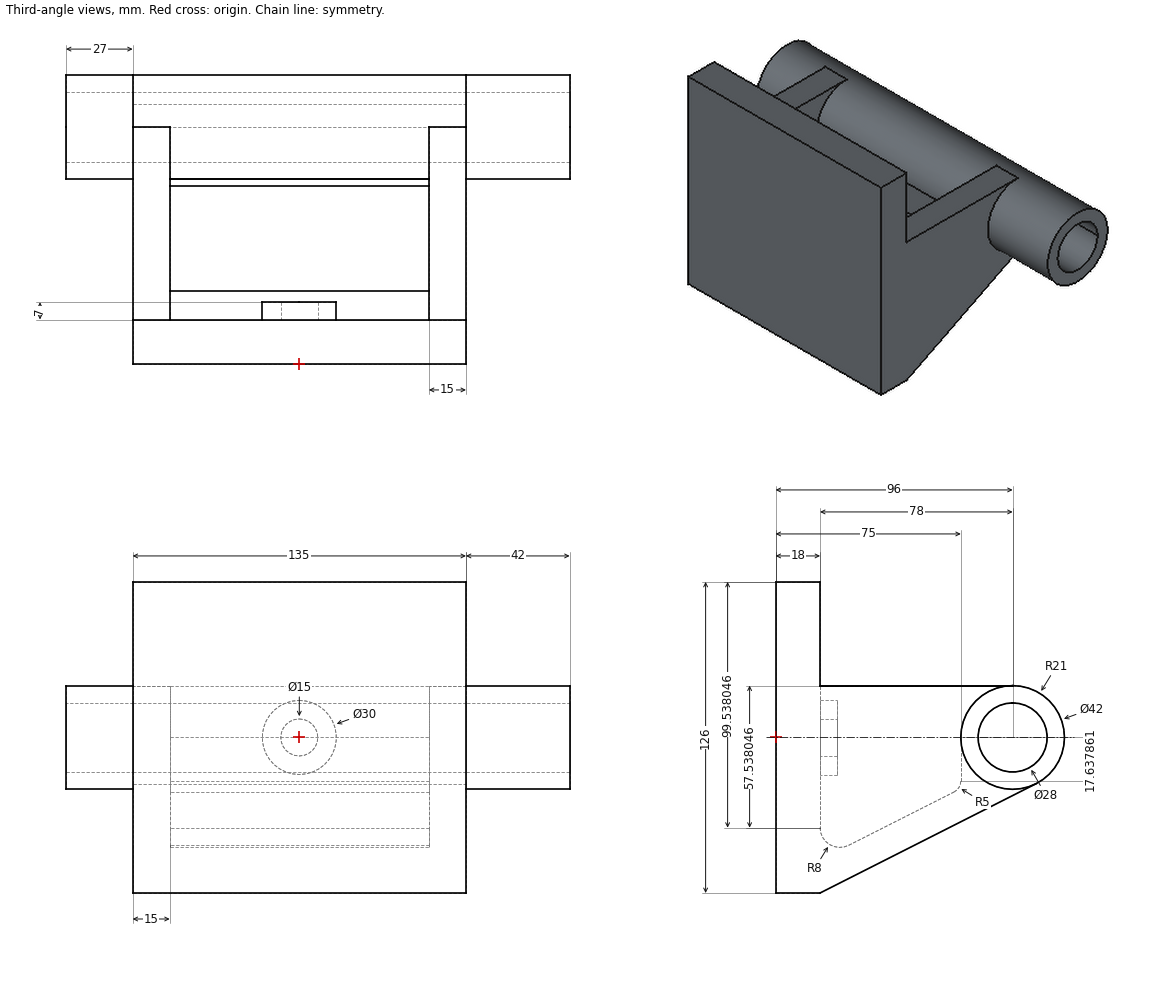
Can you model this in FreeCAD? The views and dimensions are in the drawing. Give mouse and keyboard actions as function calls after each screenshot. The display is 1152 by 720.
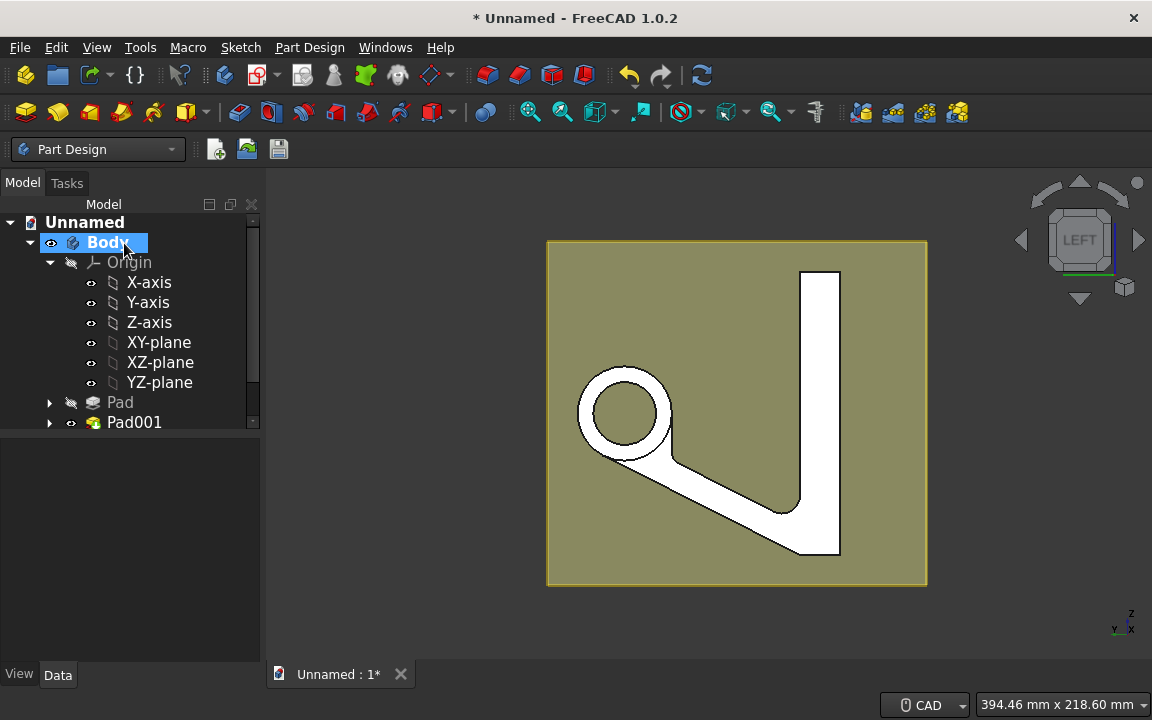
scroll(100, 318, down, 3)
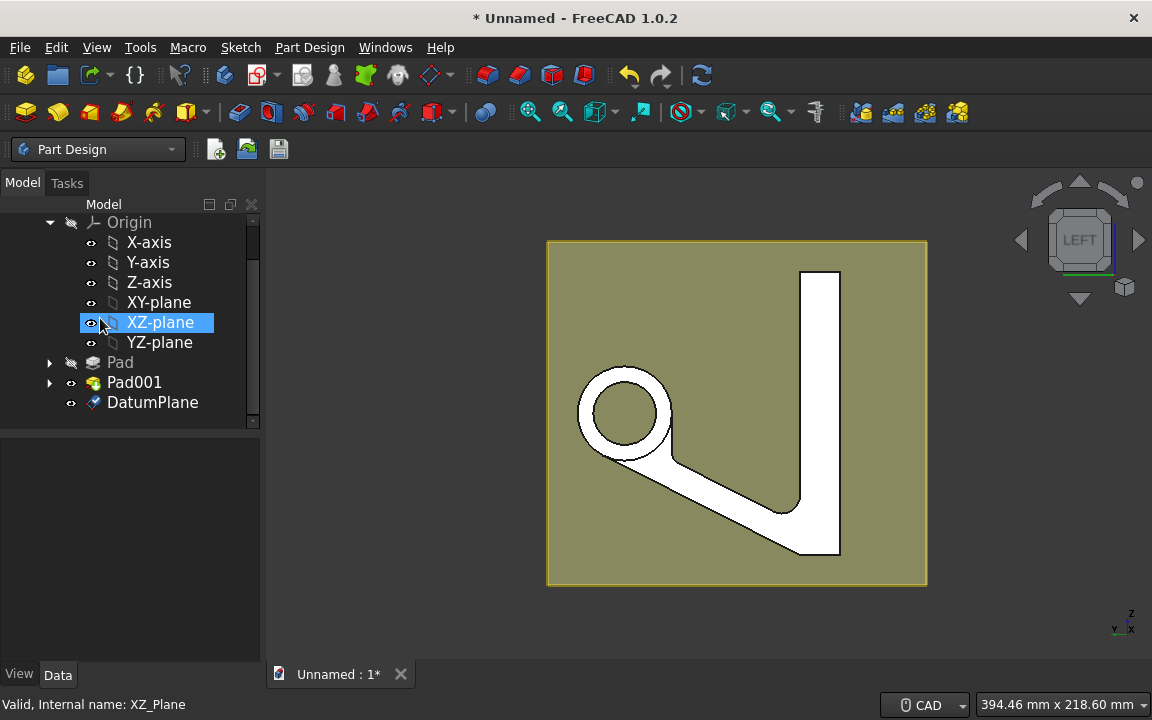
click(116, 403)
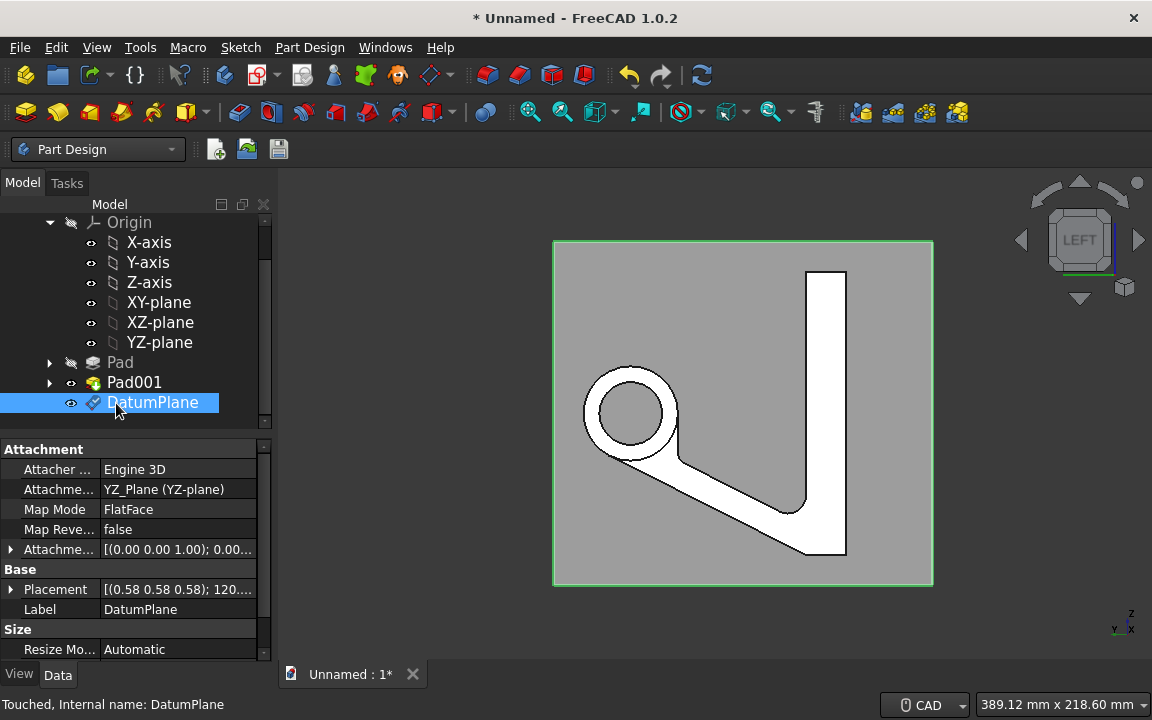
click(258, 76)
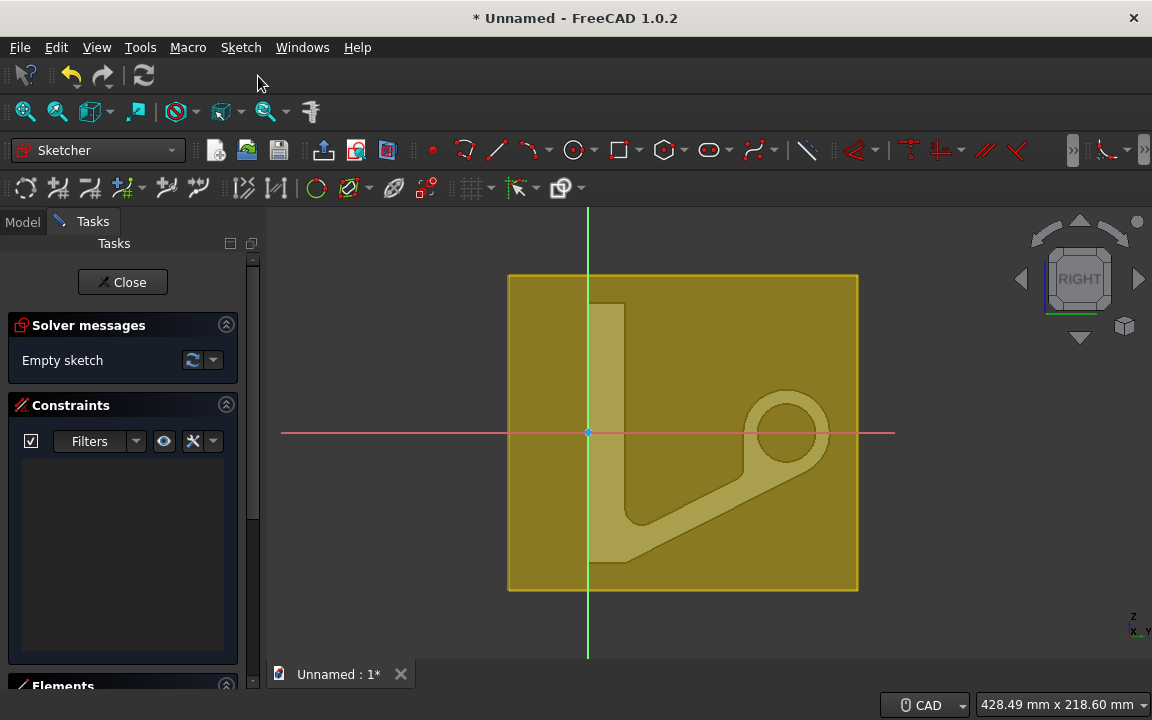
scroll(850, 433, up, 6)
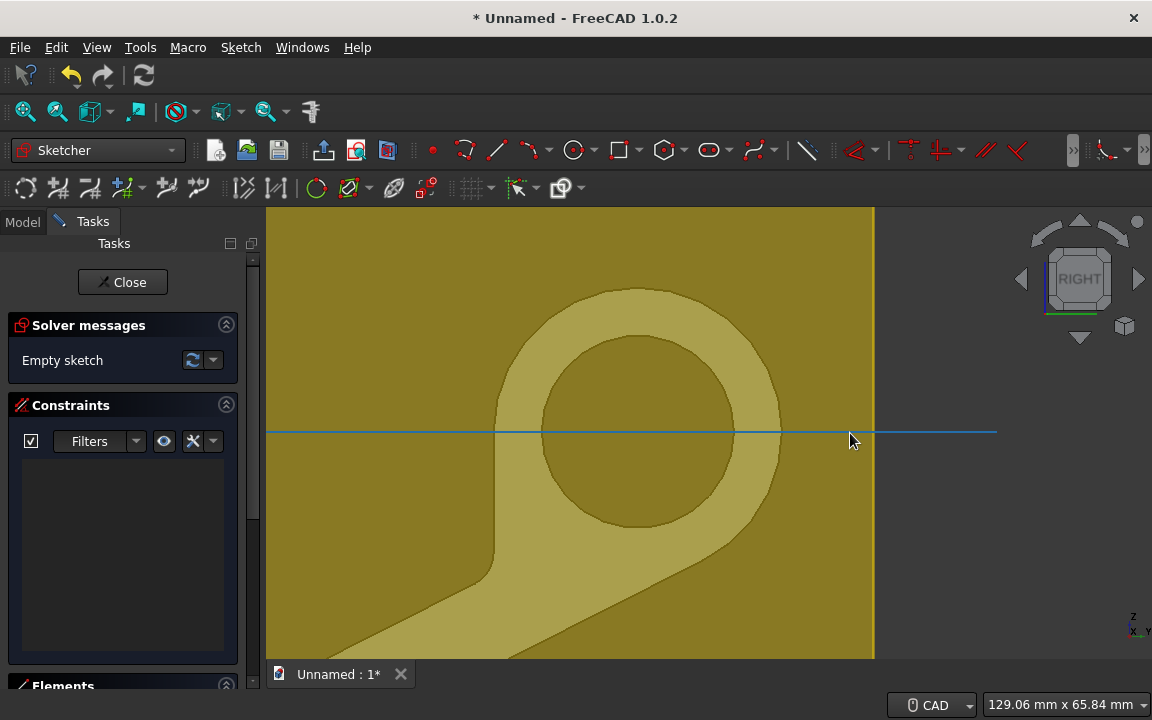
click(574, 150)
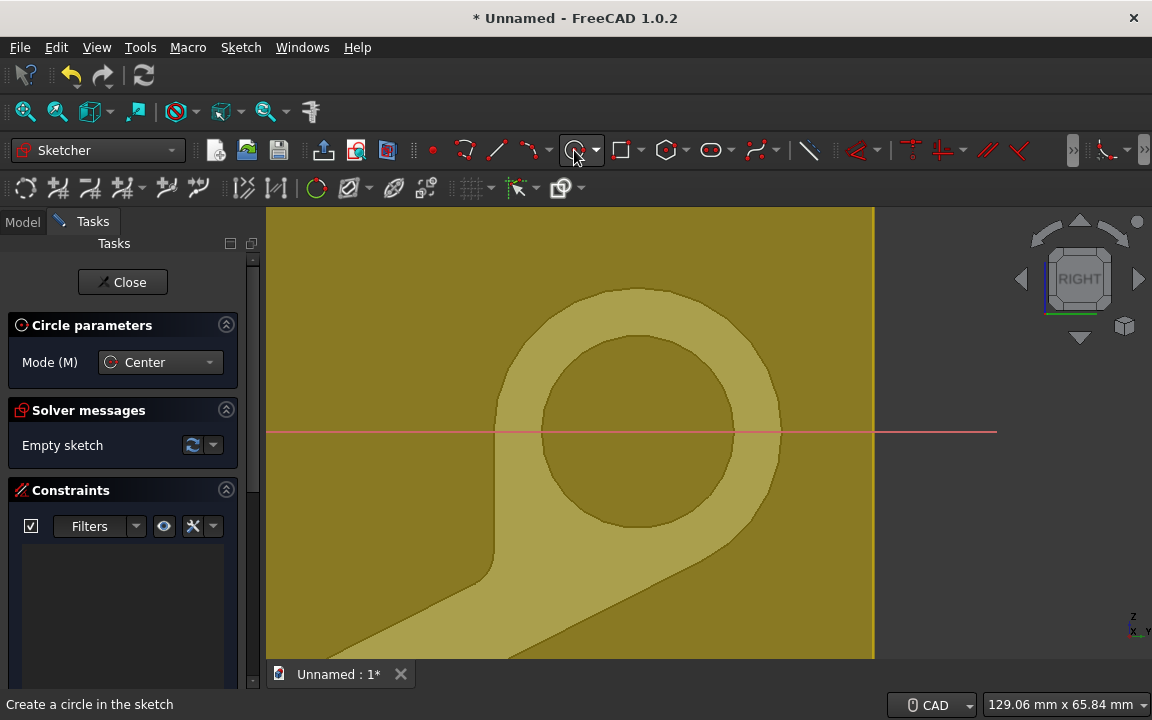
click(638, 432)
click(740, 330)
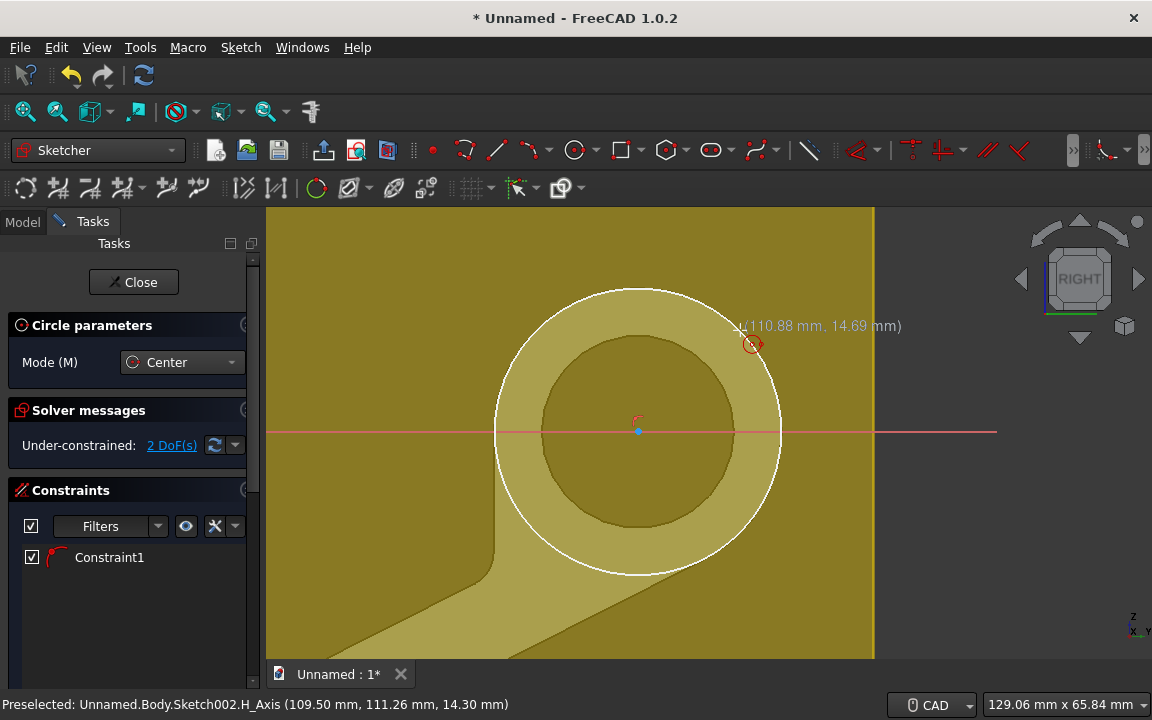
click(638, 432)
click(706, 364)
key(Escape)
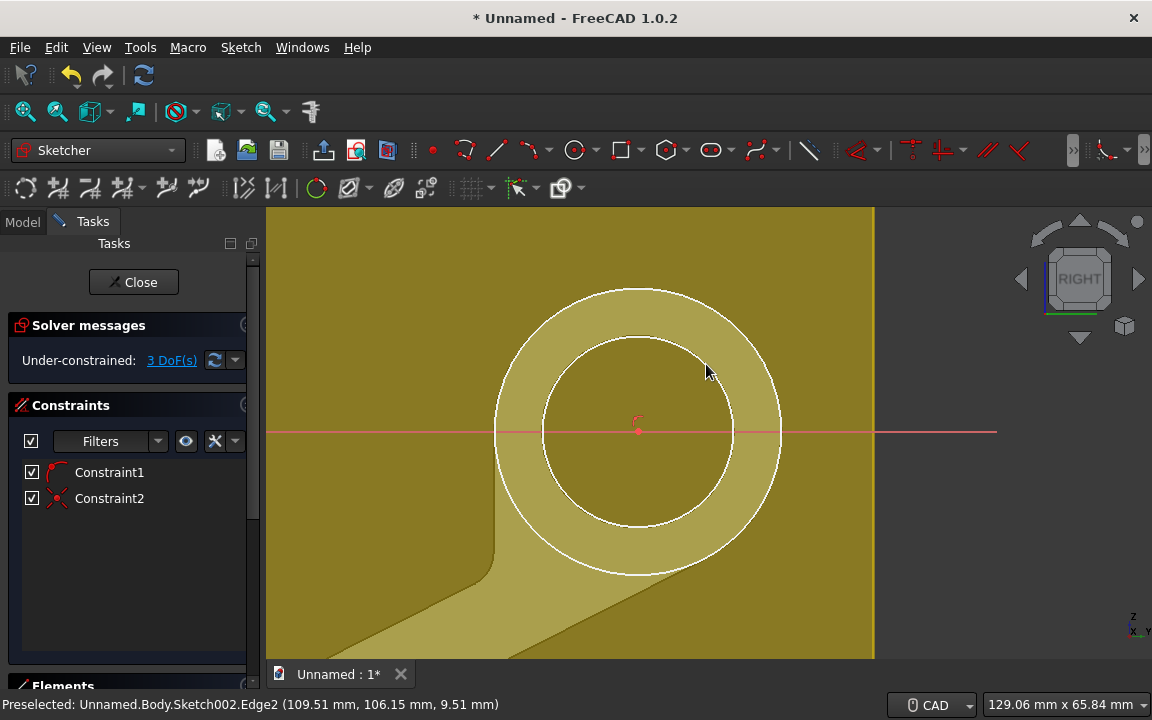
click(856, 150)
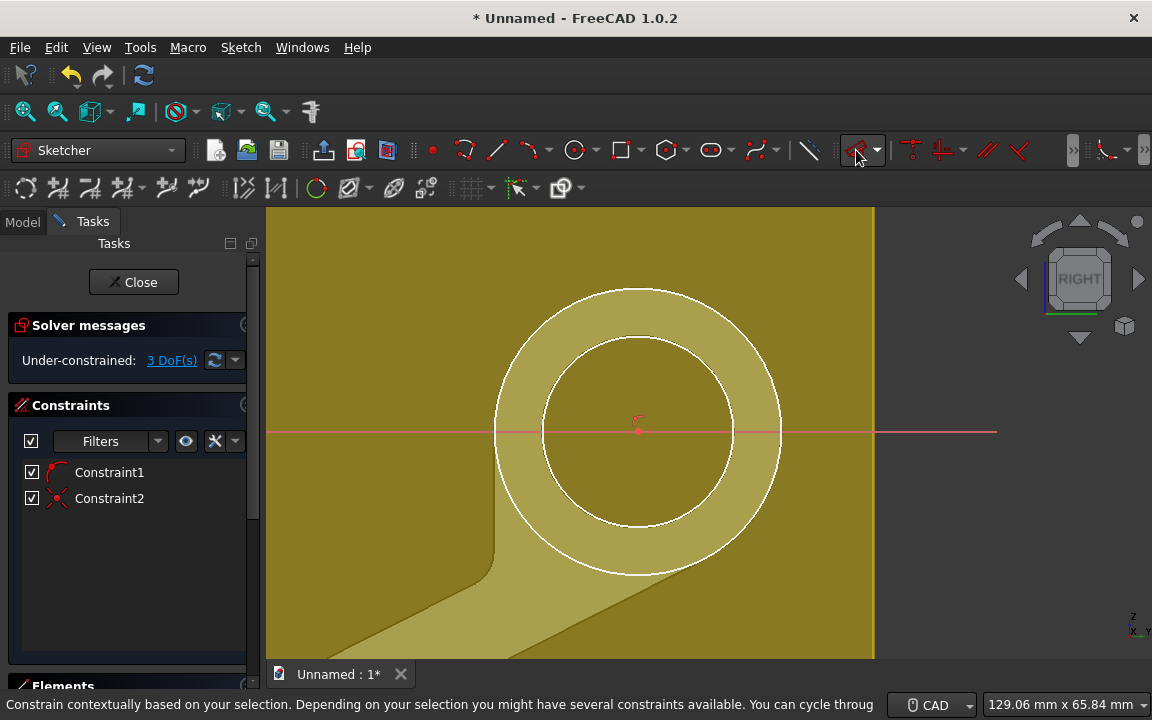
click(739, 330)
click(762, 307)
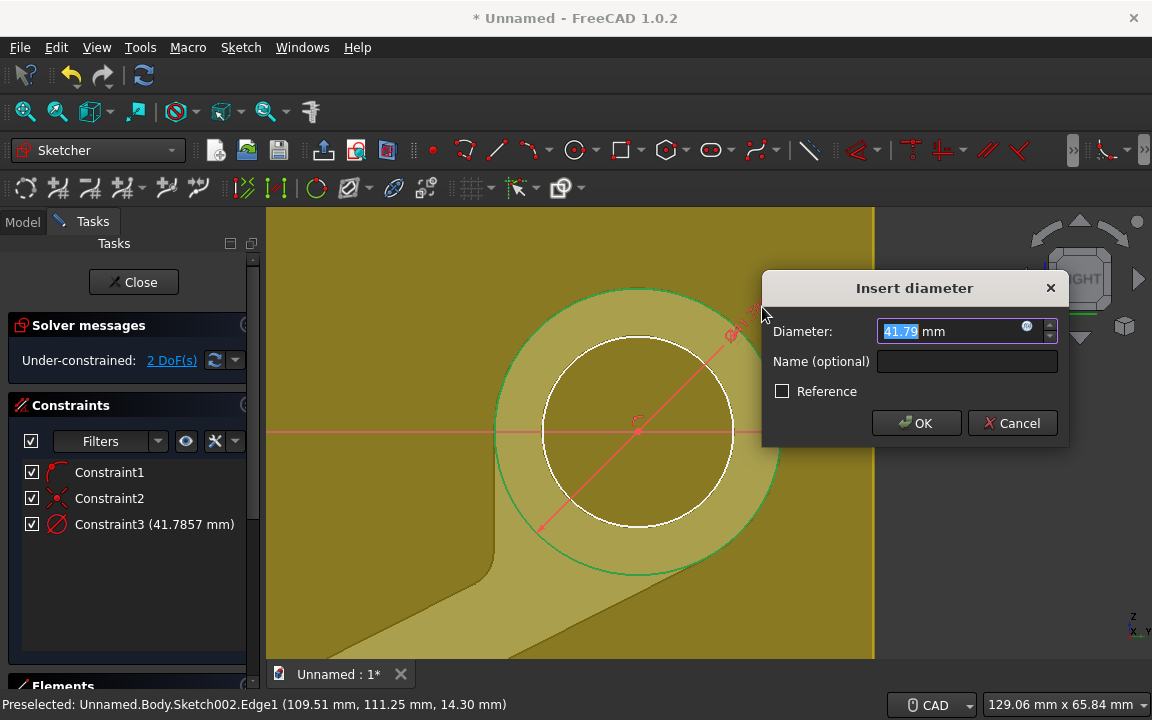
text(42)
key(Return)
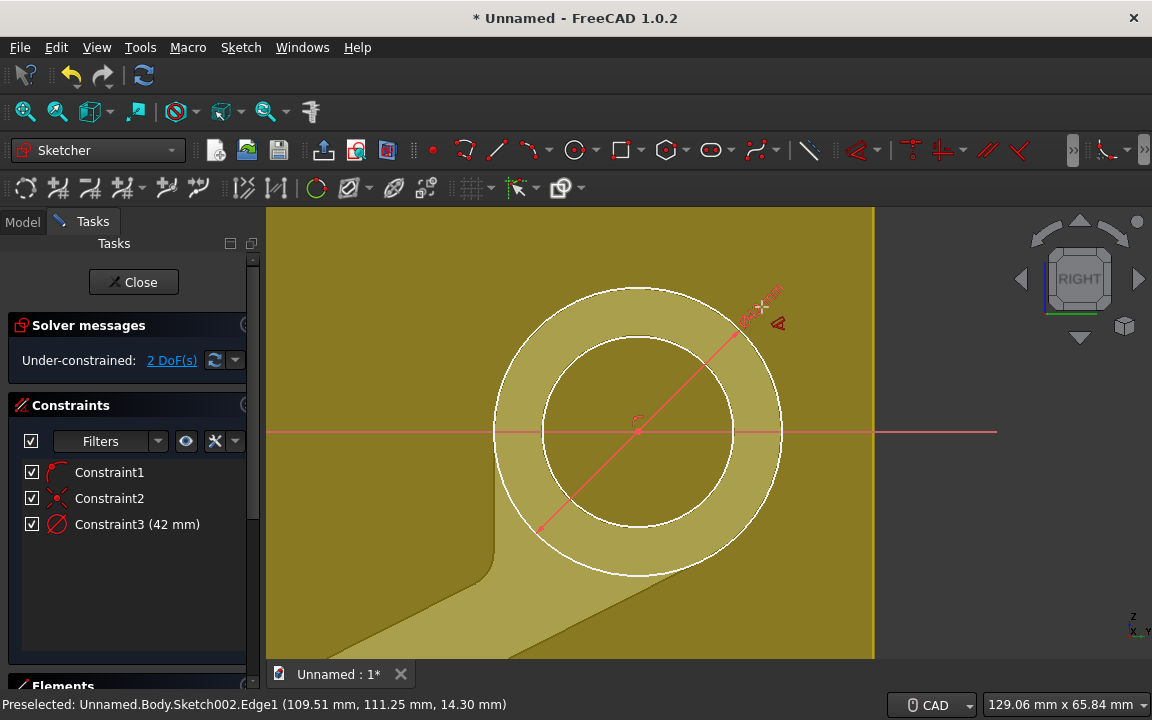
click(705, 364)
click(727, 341)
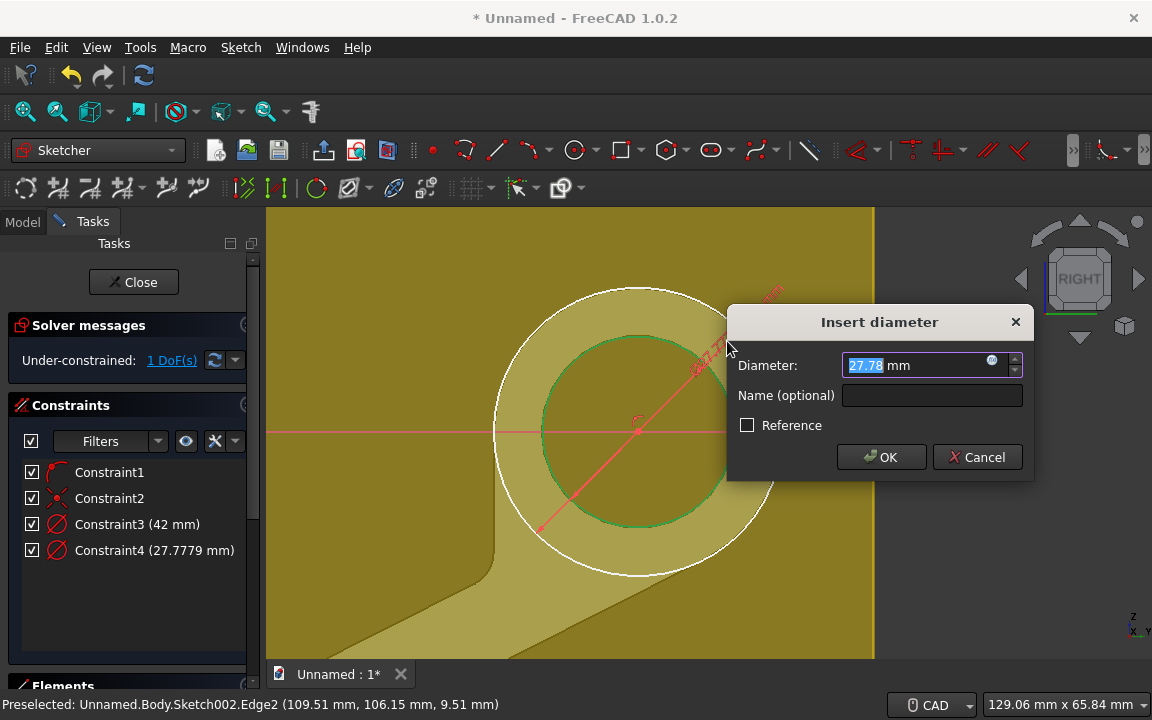
text(28)
key(Return)